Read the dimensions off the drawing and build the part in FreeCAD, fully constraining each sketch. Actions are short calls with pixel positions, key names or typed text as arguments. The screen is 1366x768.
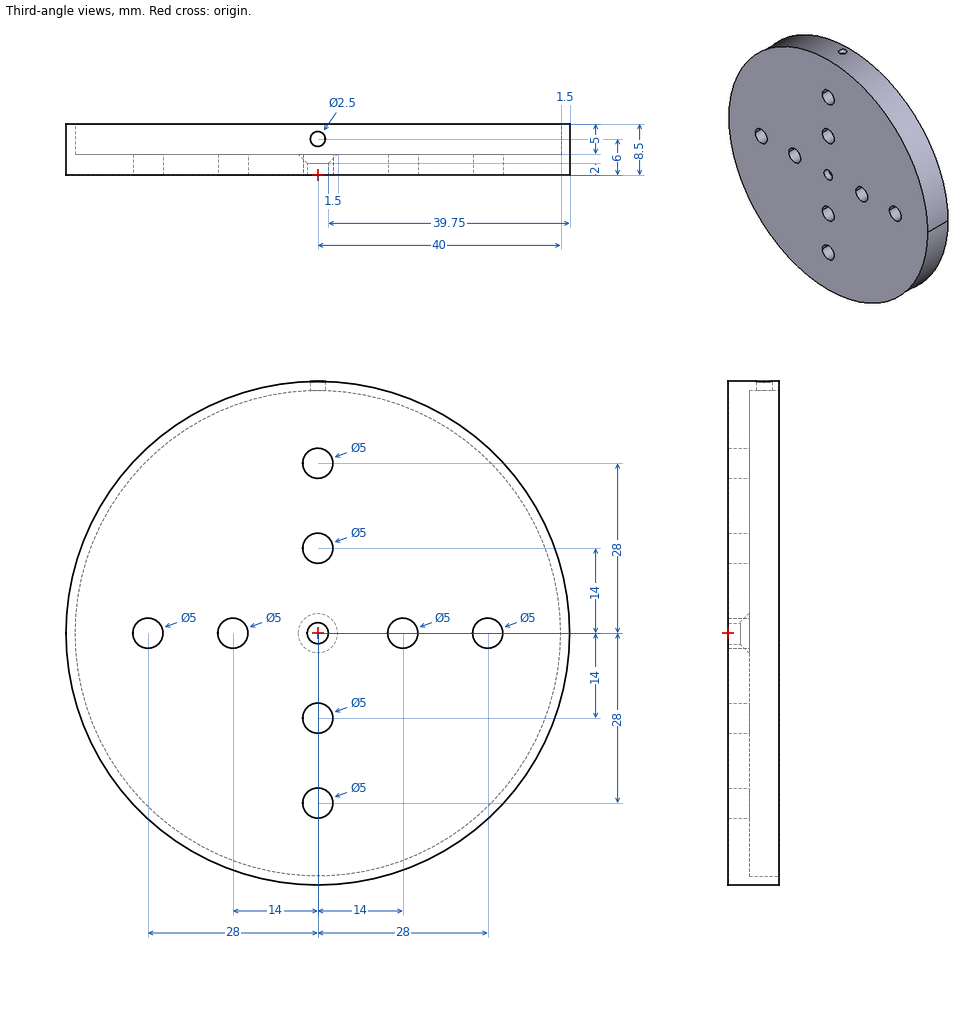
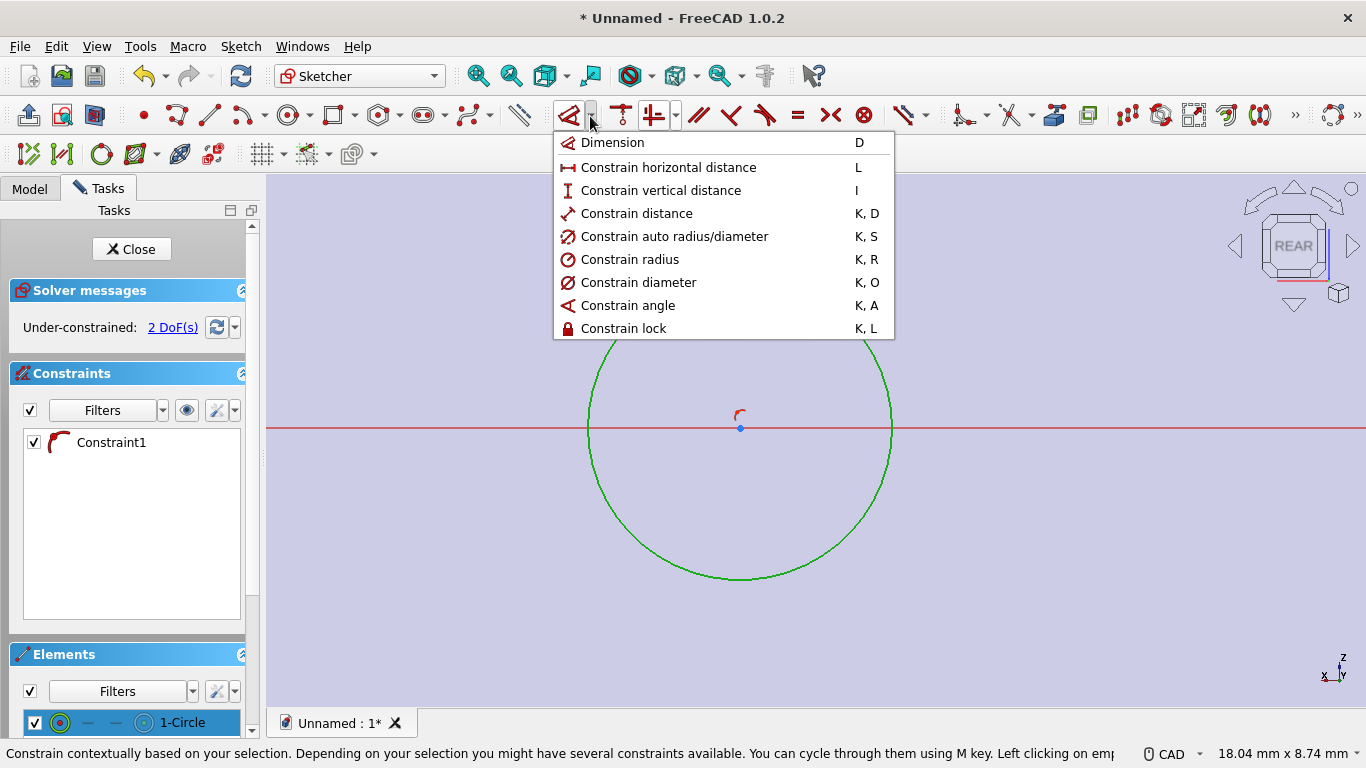
click(724, 282)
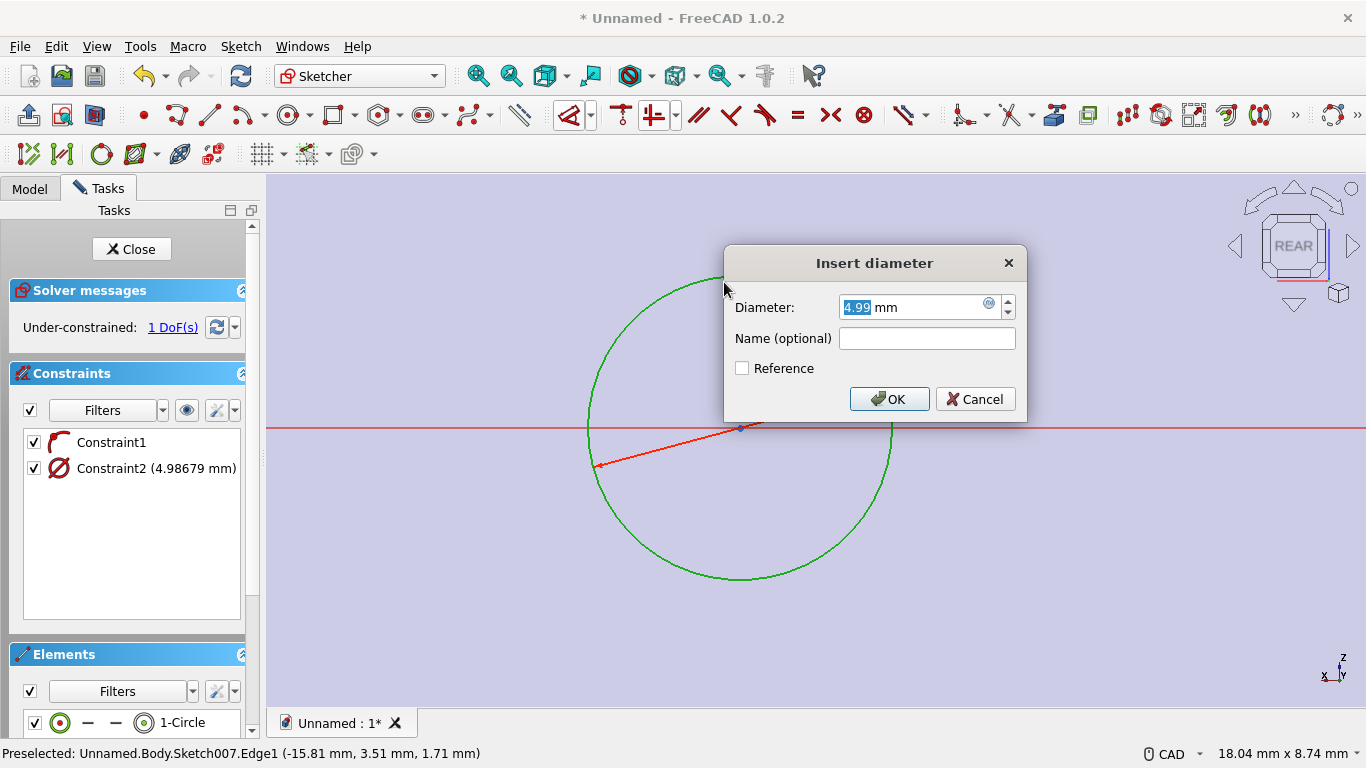
text(5)
key(Return)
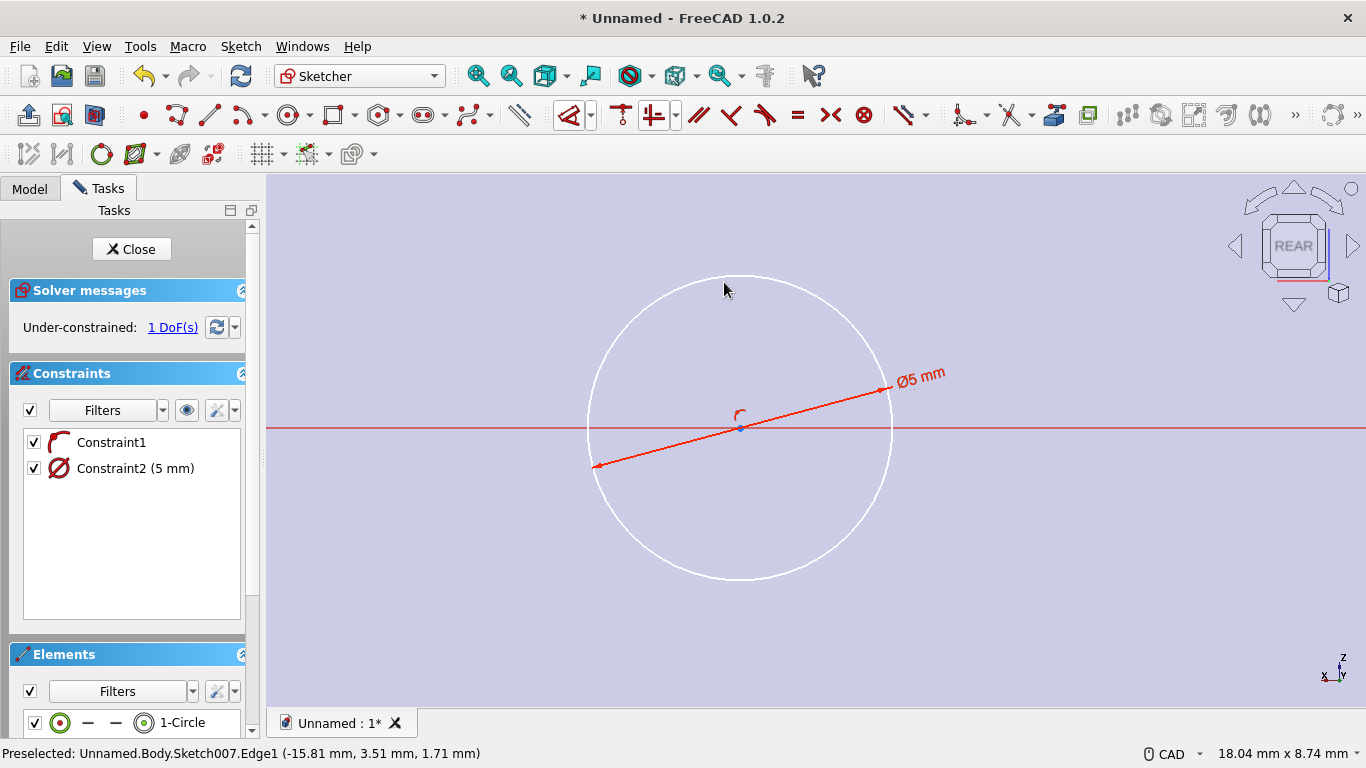
click(740, 428)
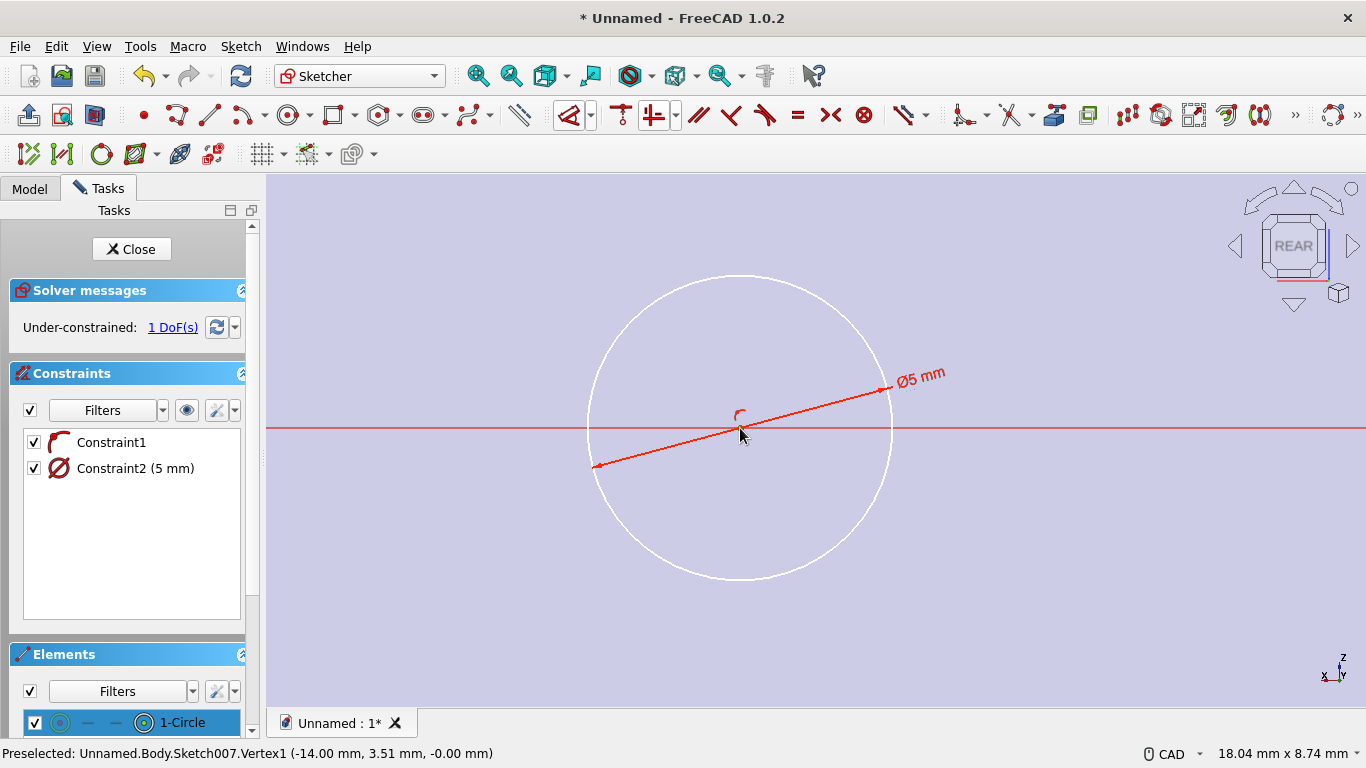
click(590, 116)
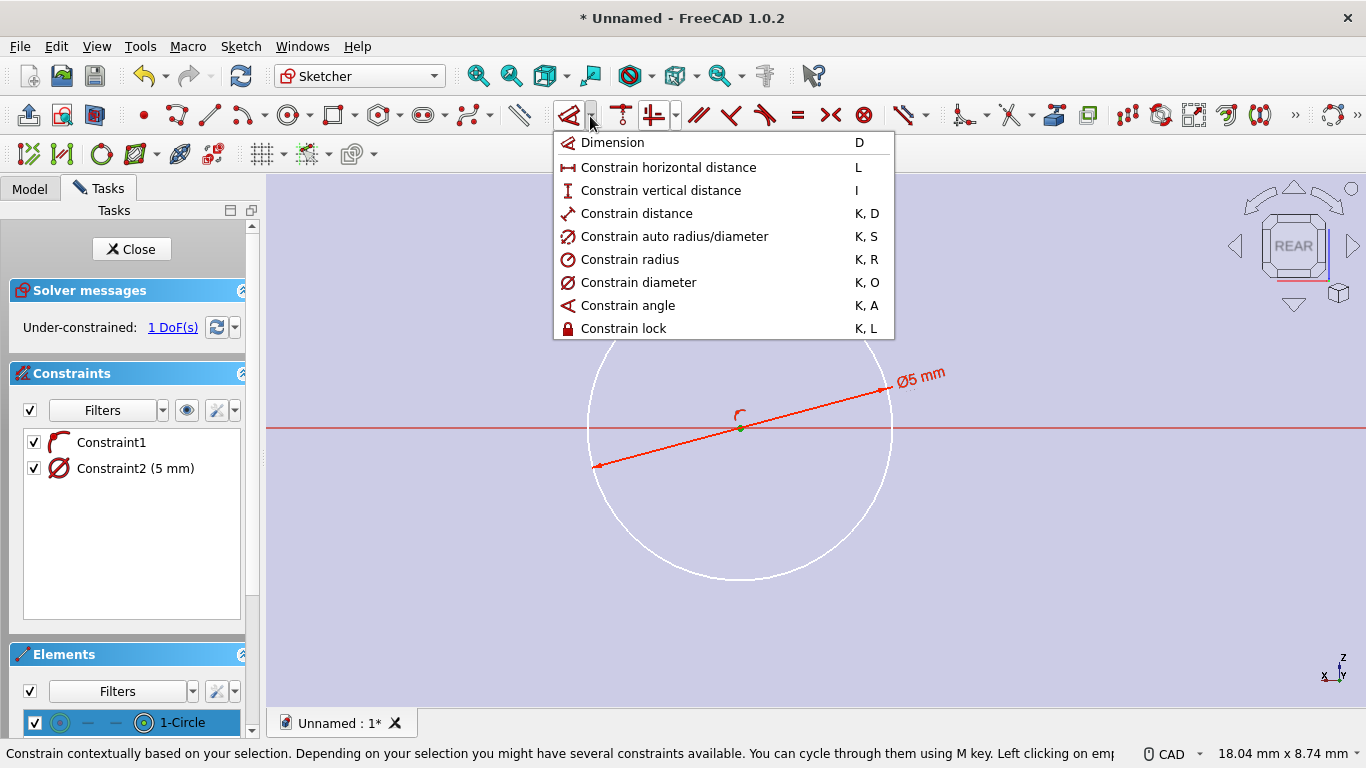
click(724, 168)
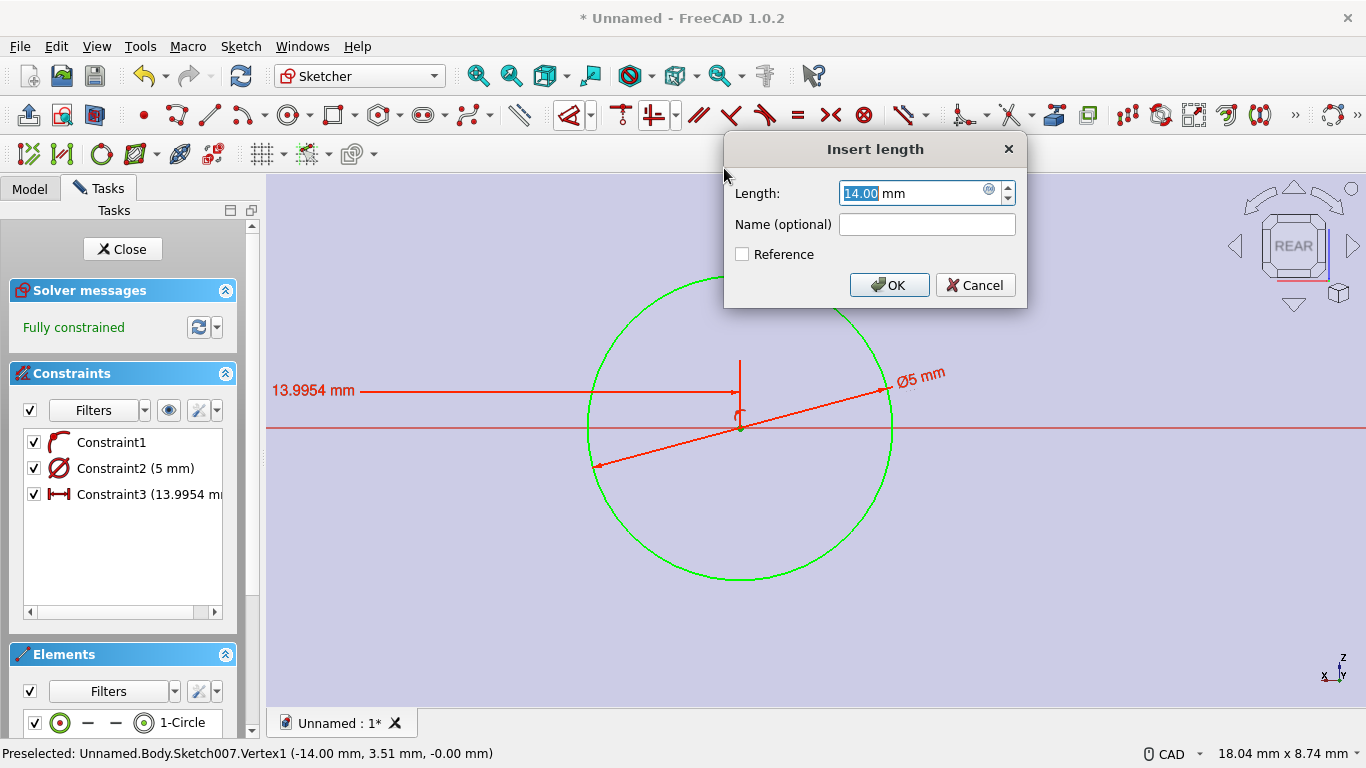
text(14)
key(Return)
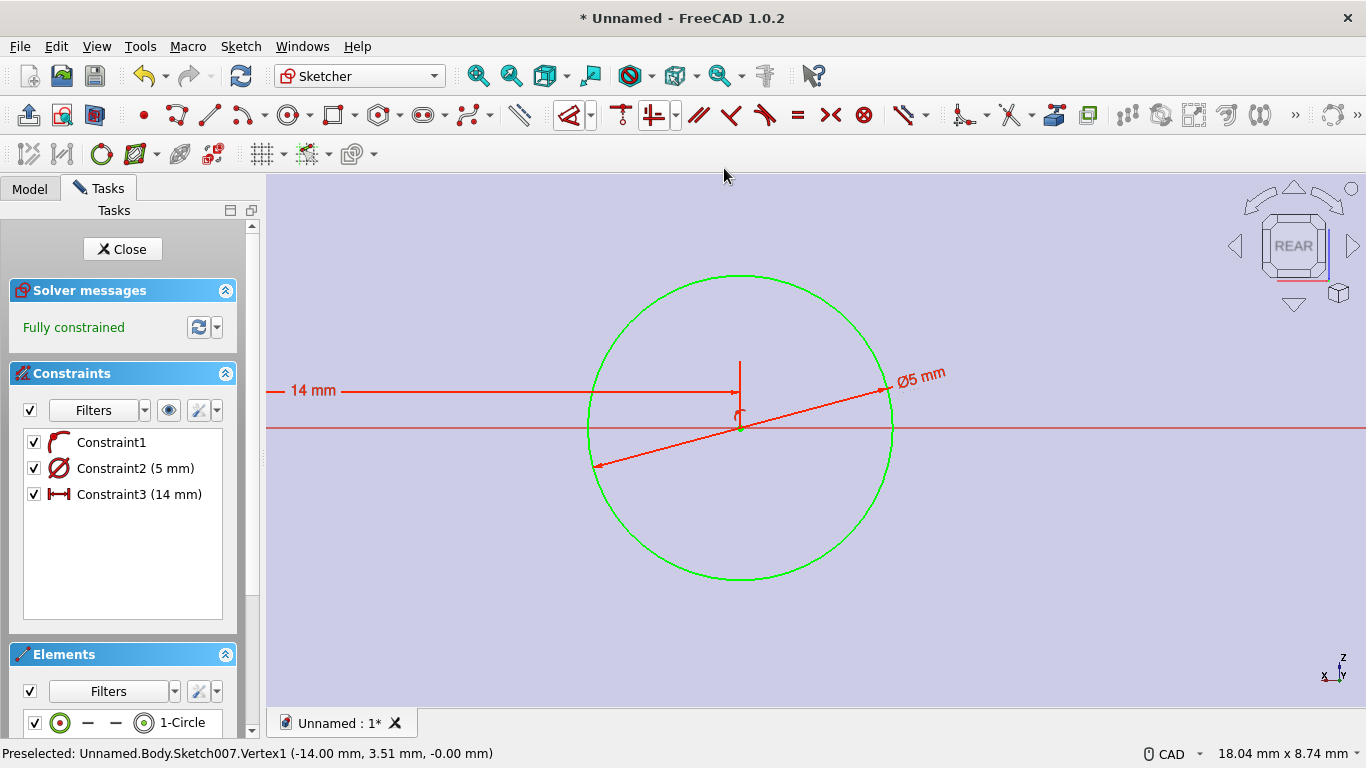
click(123, 249)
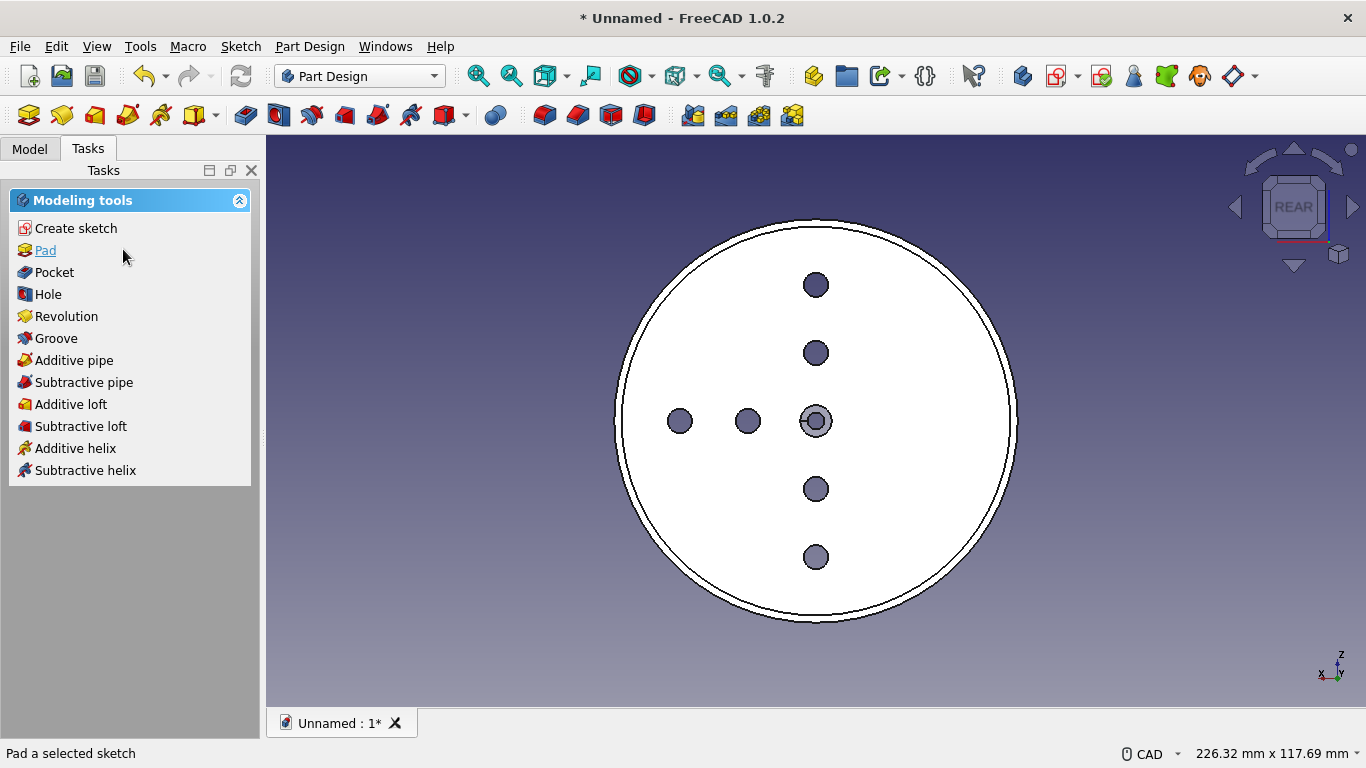
click(246, 116)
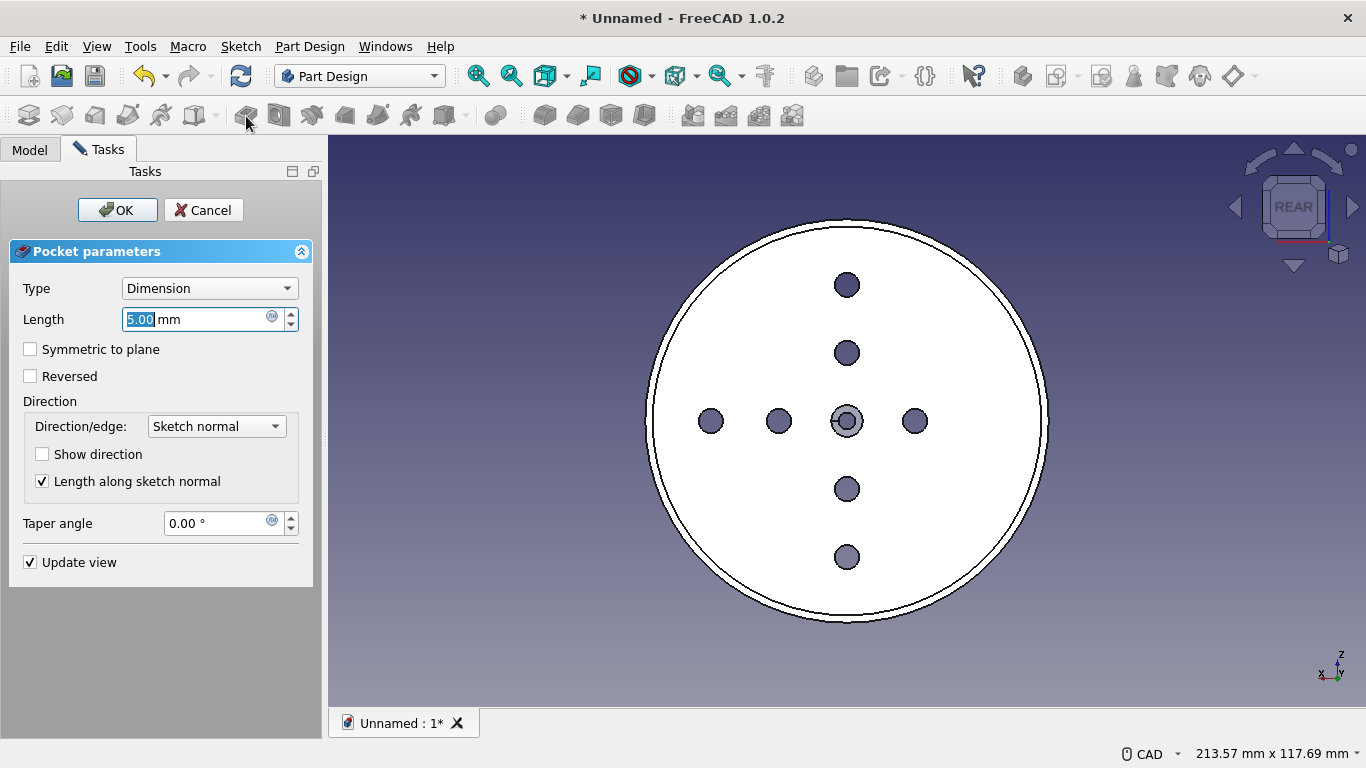
click(210, 288)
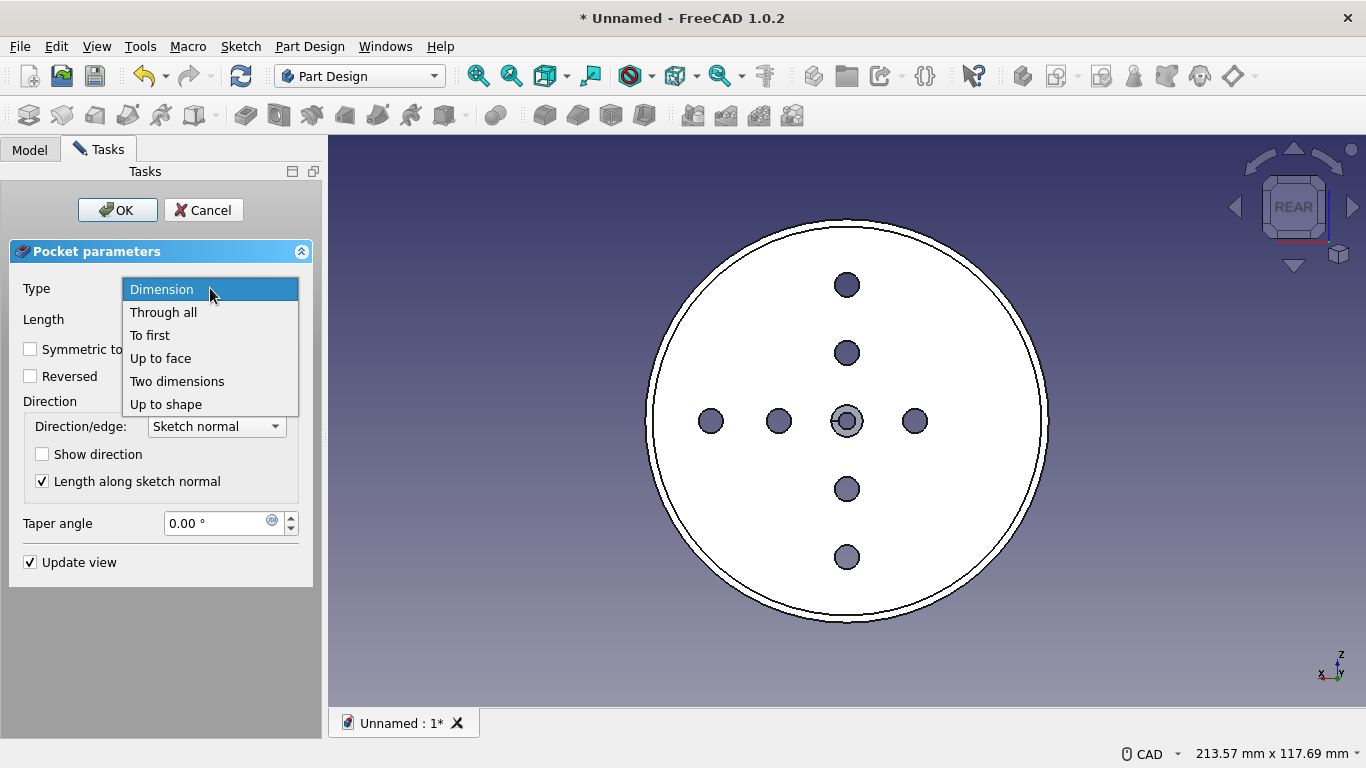
click(208, 336)